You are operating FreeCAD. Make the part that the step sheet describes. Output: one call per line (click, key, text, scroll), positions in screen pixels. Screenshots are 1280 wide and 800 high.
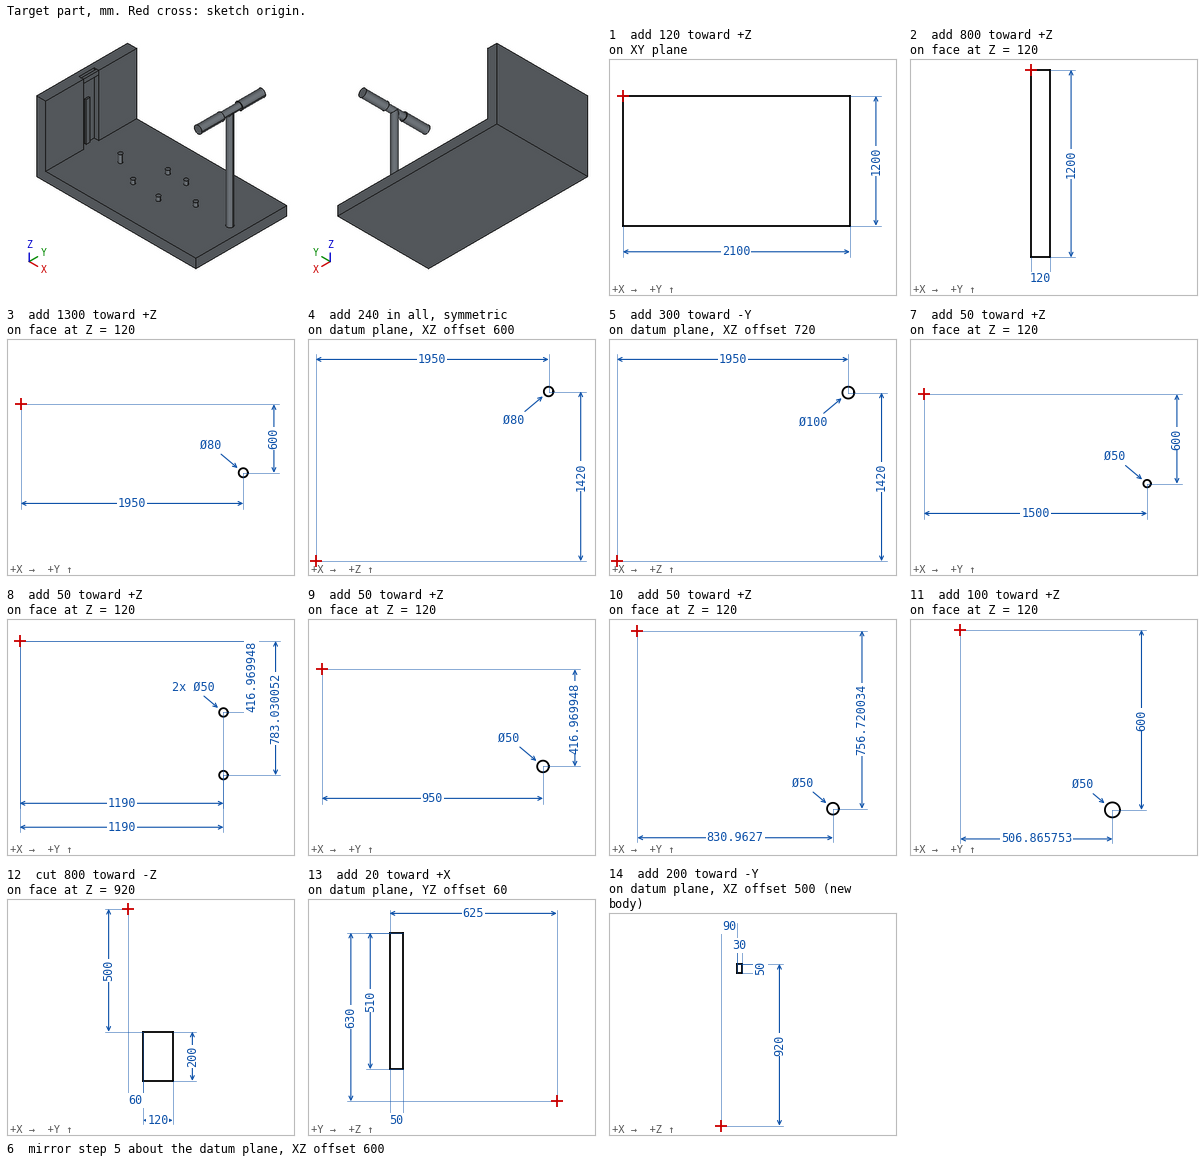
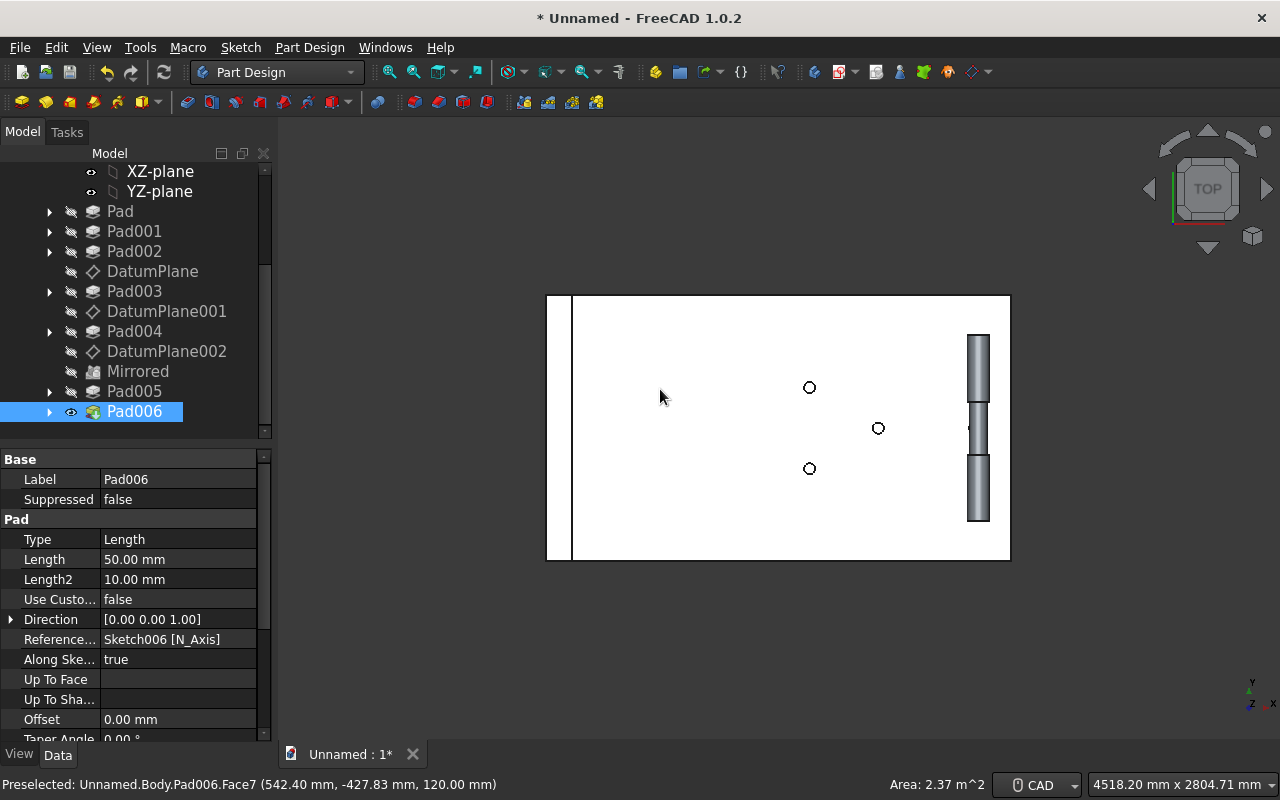
click(840, 72)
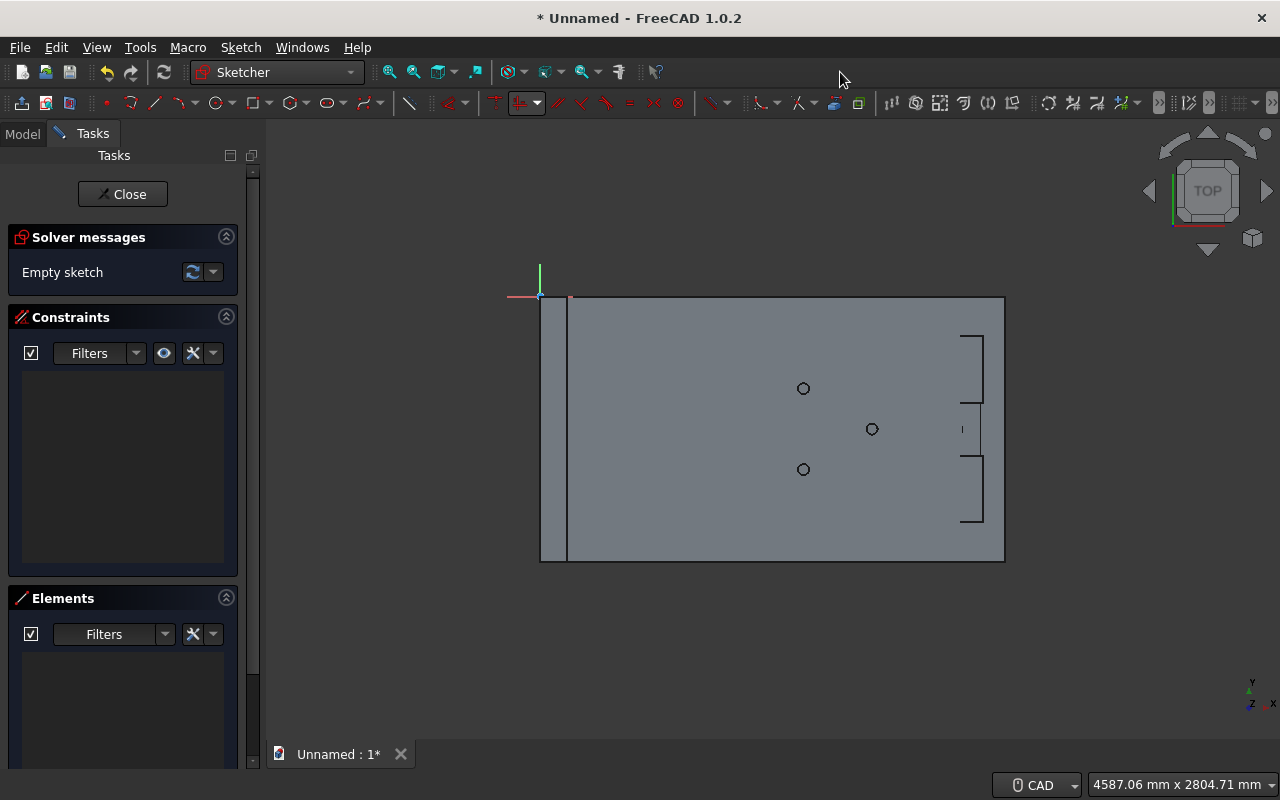
click(70, 104)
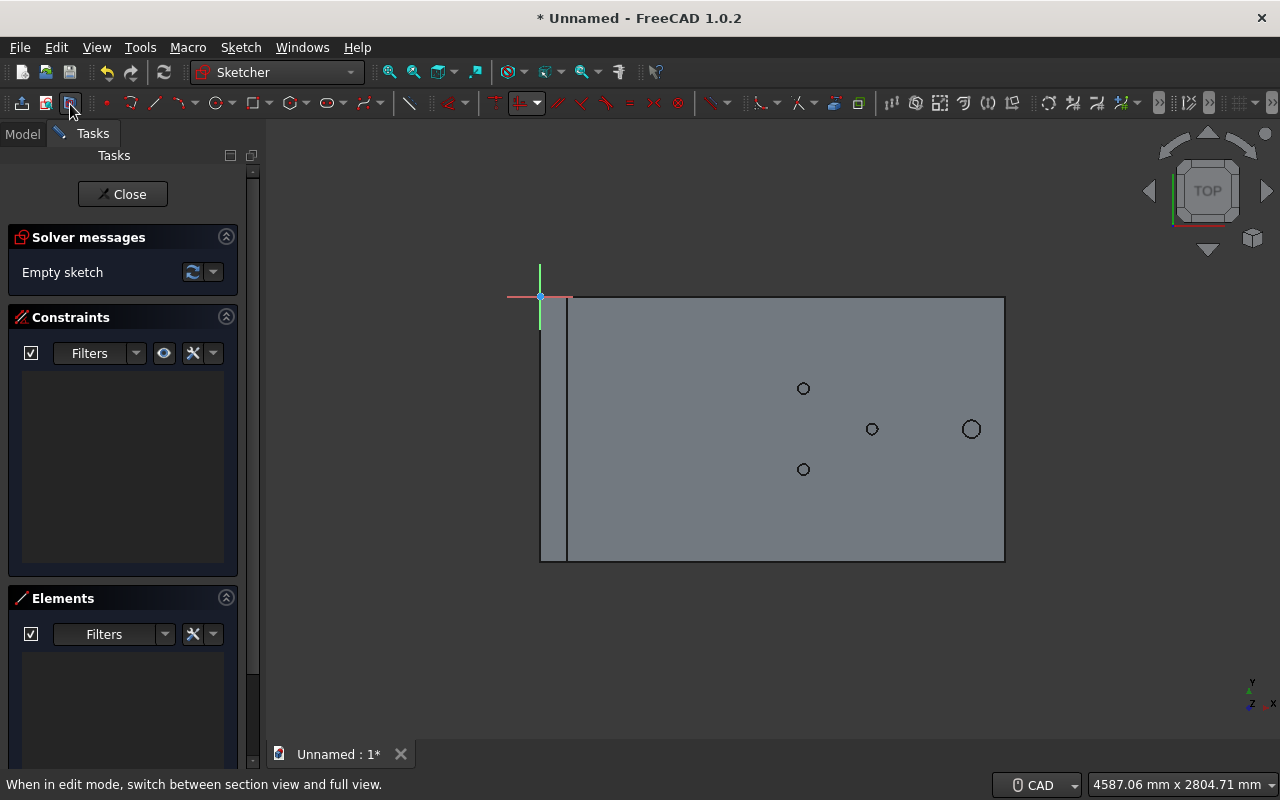
scroll(753, 387, up, 15)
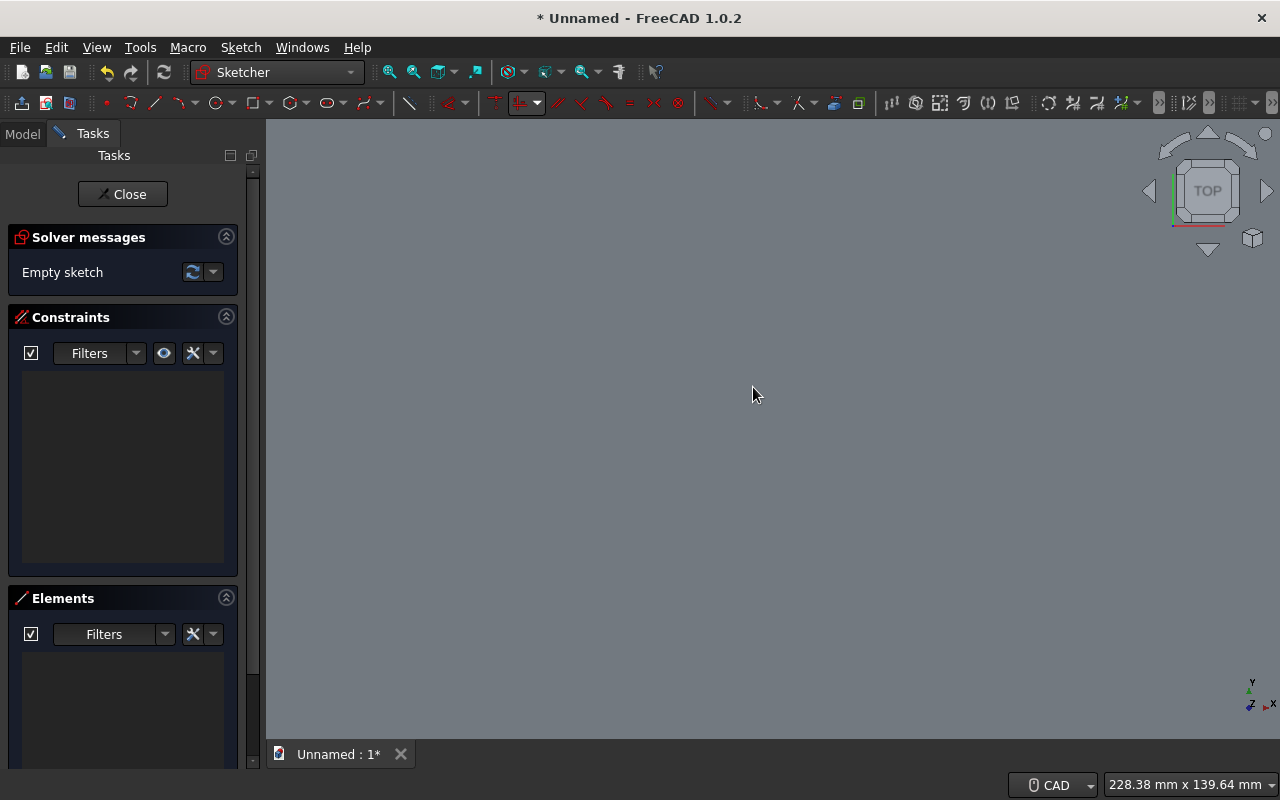
scroll(679, 394, up, 3)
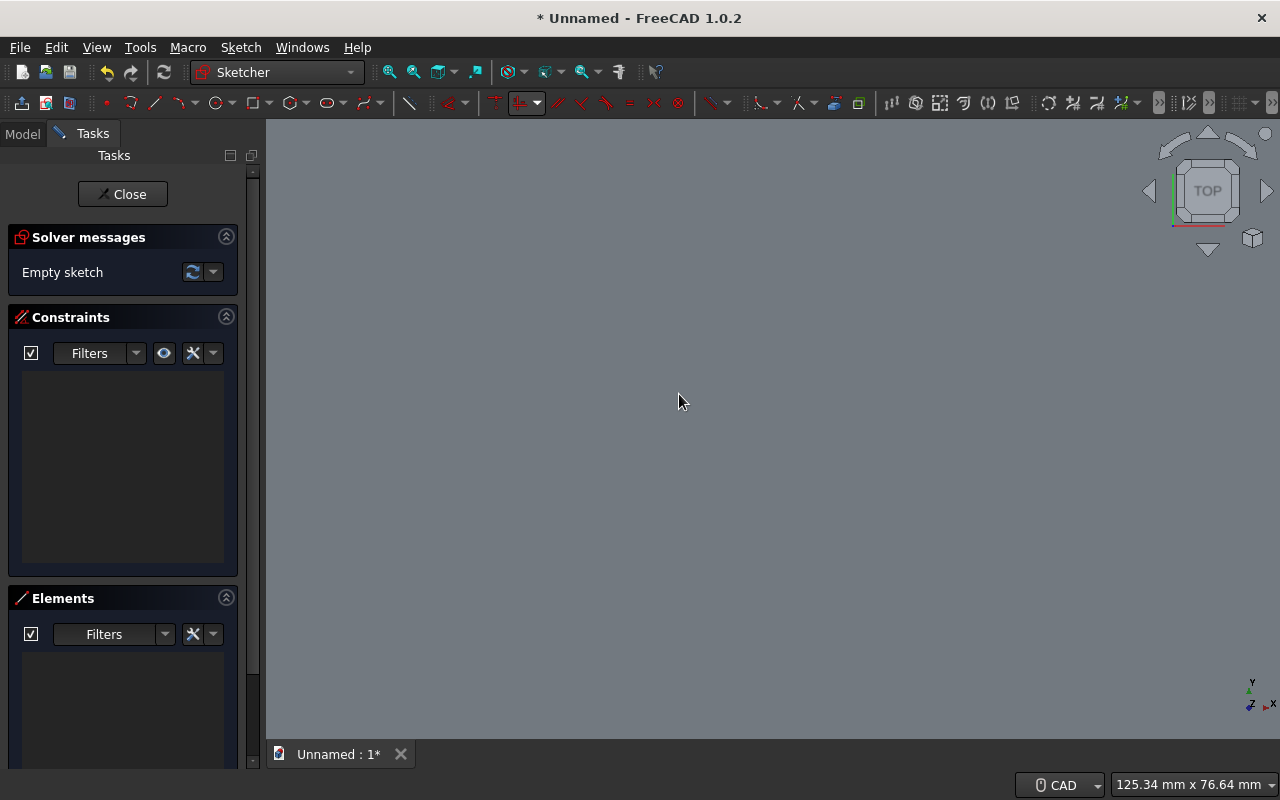
click(216, 104)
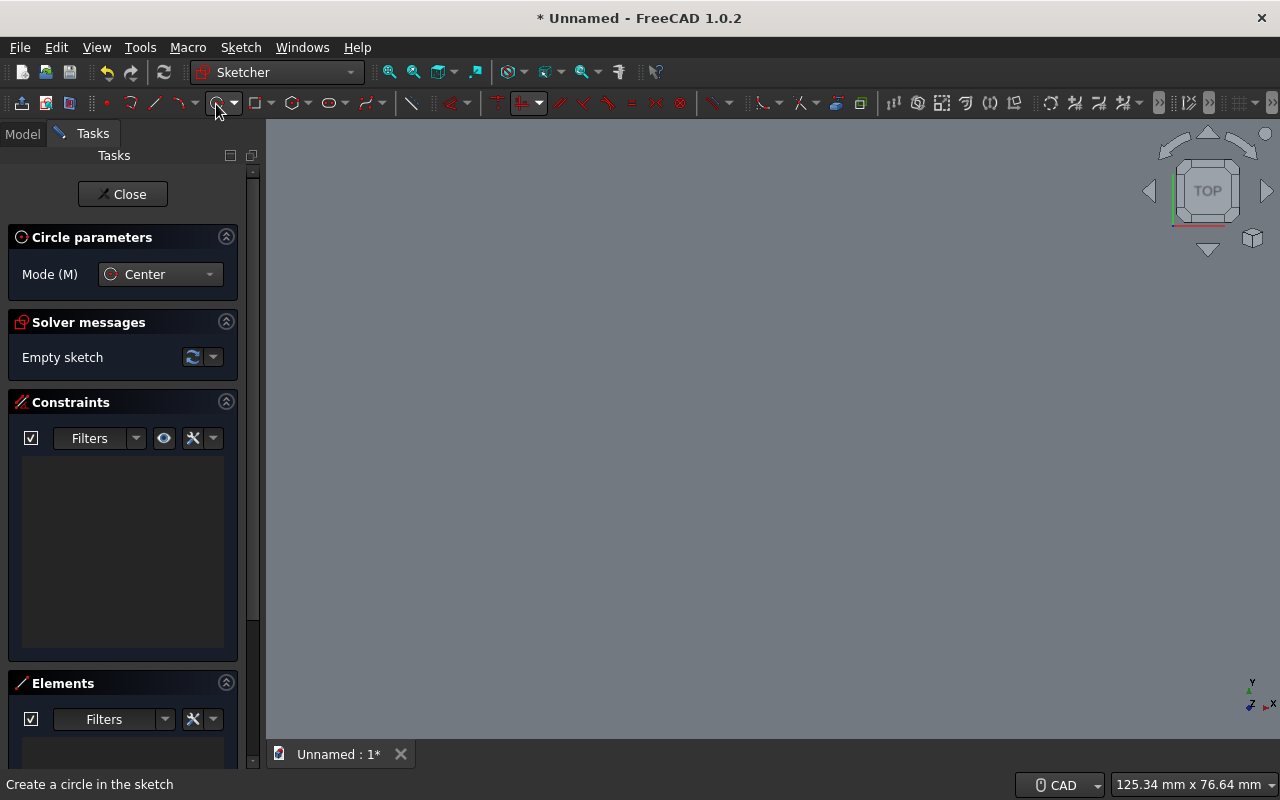
click(704, 429)
move(847, 286)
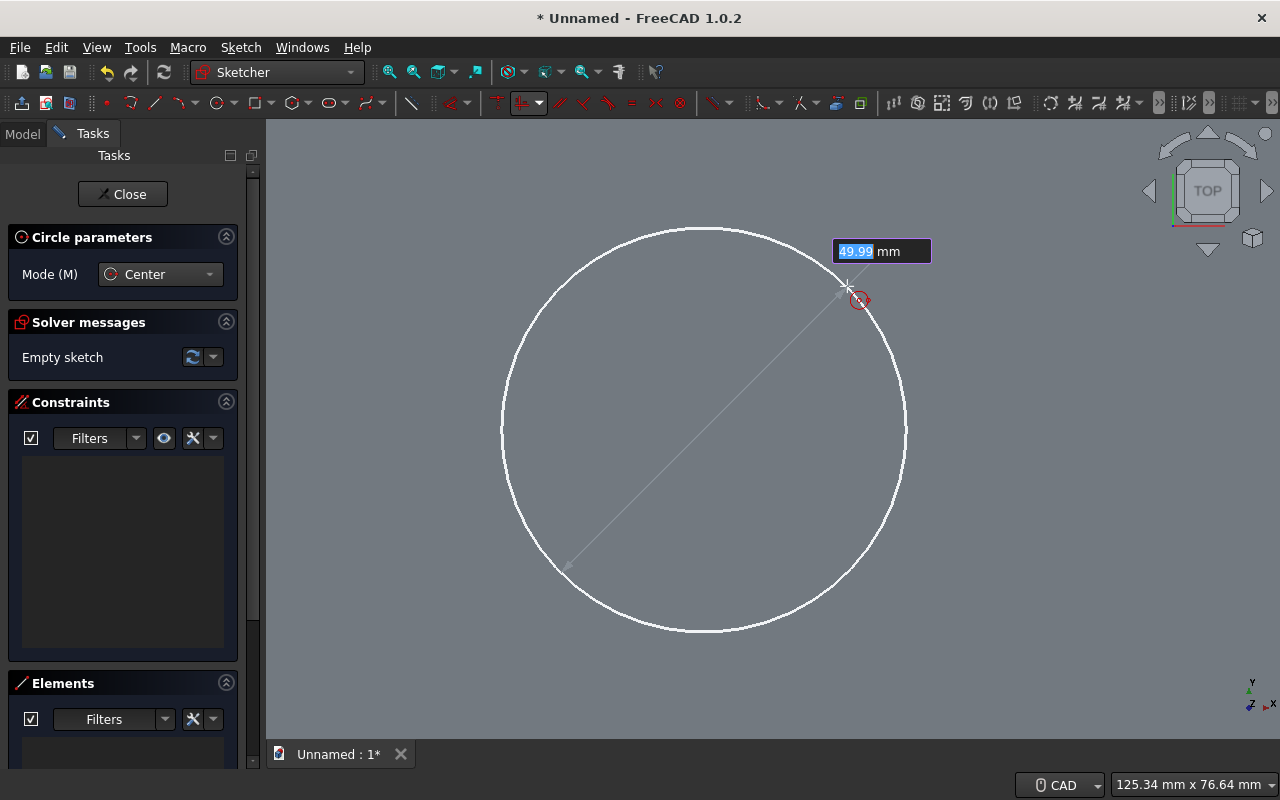
text(50)
key(Return)
key(Escape)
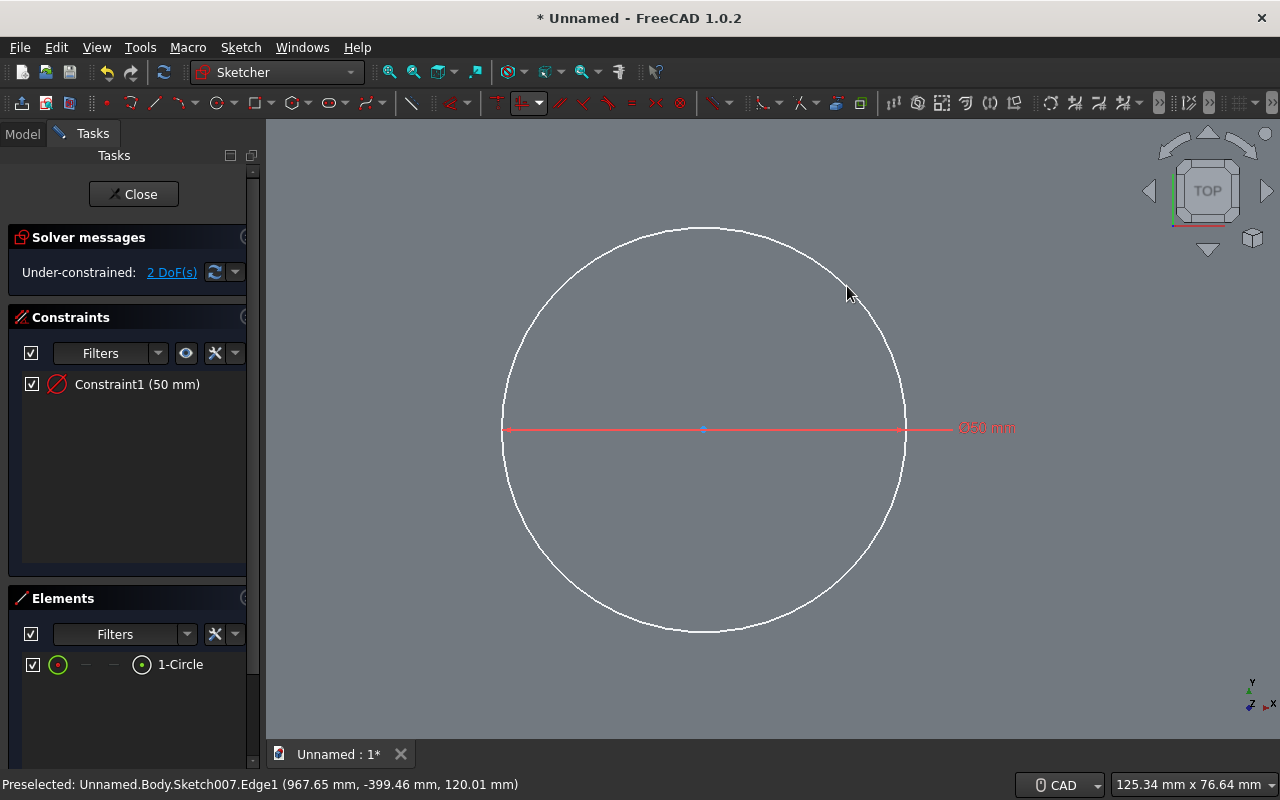
key(d)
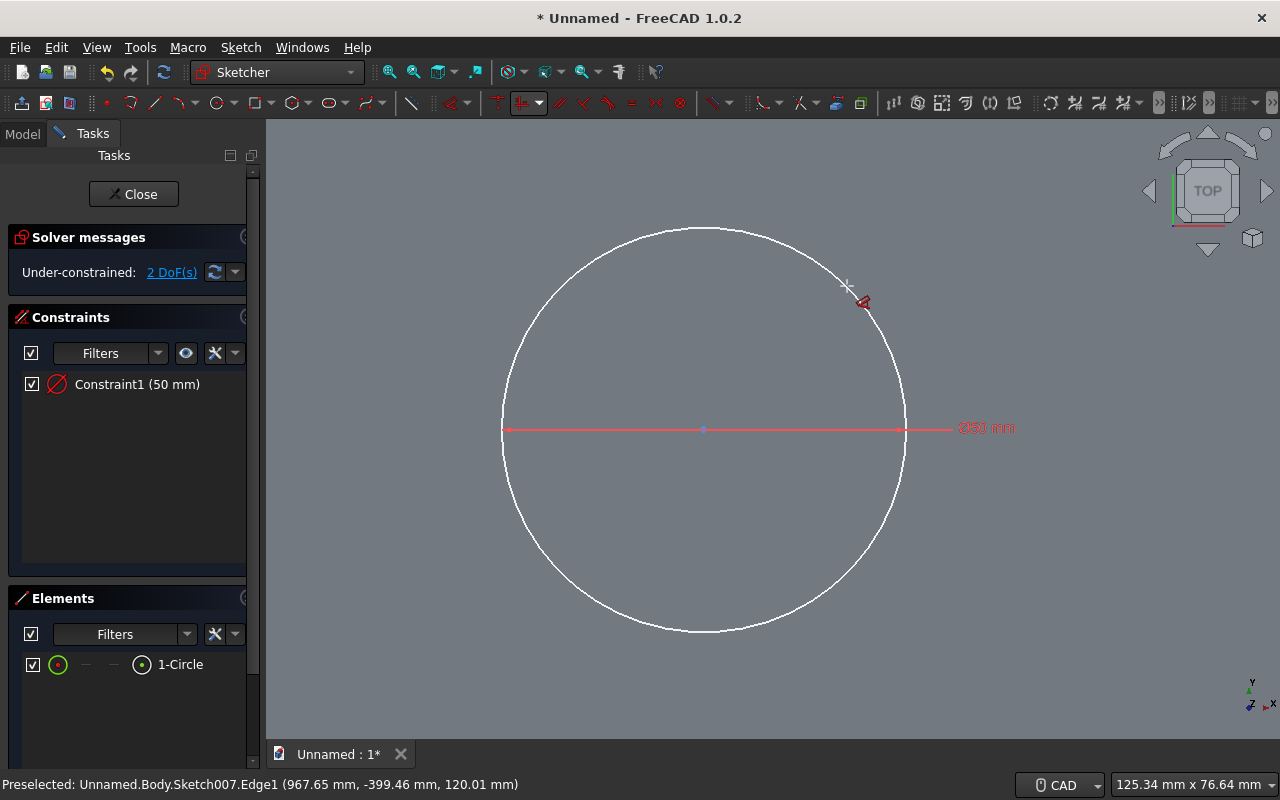
click(704, 430)
click(405, 464)